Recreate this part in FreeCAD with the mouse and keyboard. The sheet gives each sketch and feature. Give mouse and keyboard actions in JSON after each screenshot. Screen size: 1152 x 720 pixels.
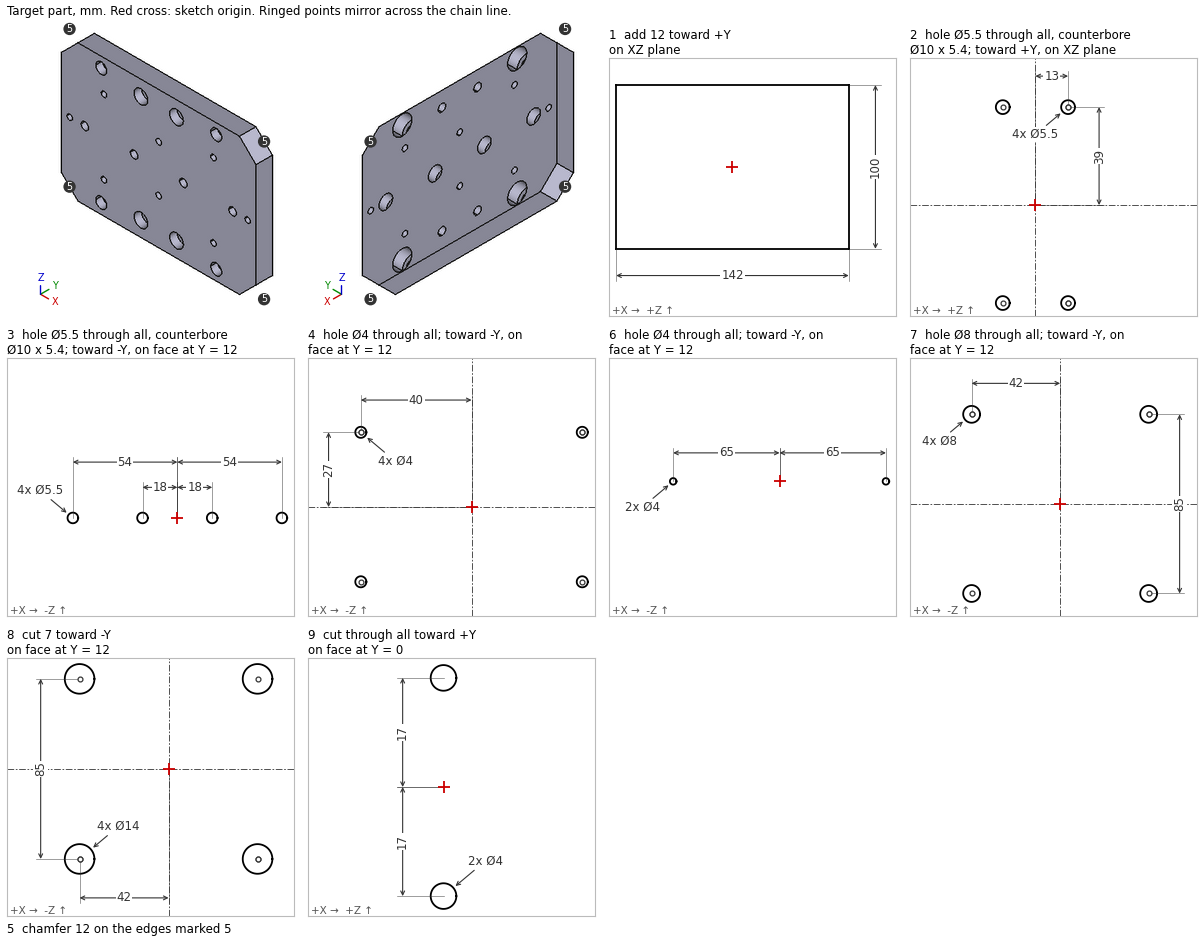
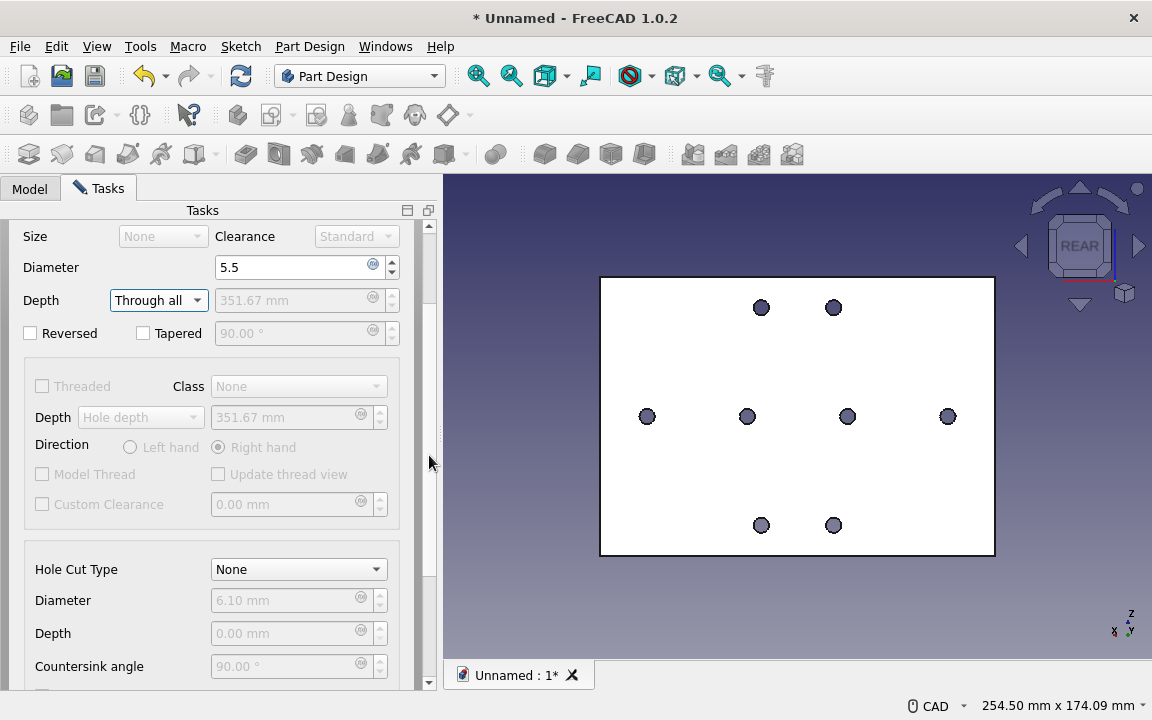
{"action": "left_click", "coordinate": [300, 570]}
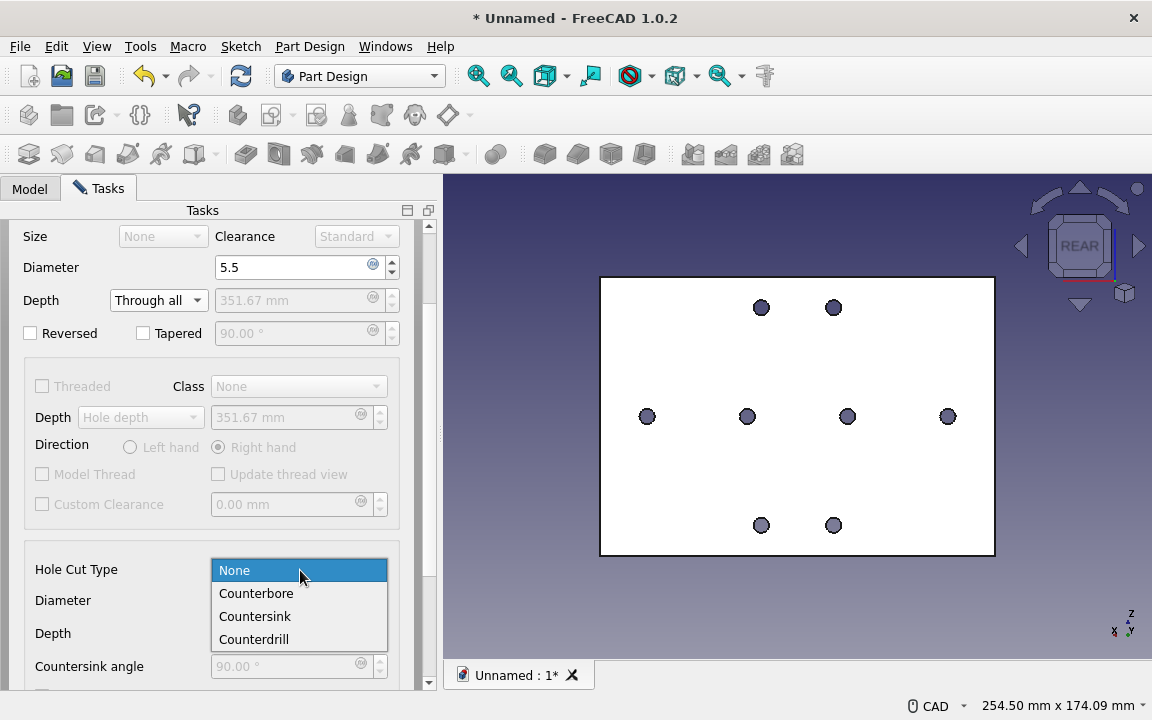
{"action": "left_click", "coordinate": [298, 594]}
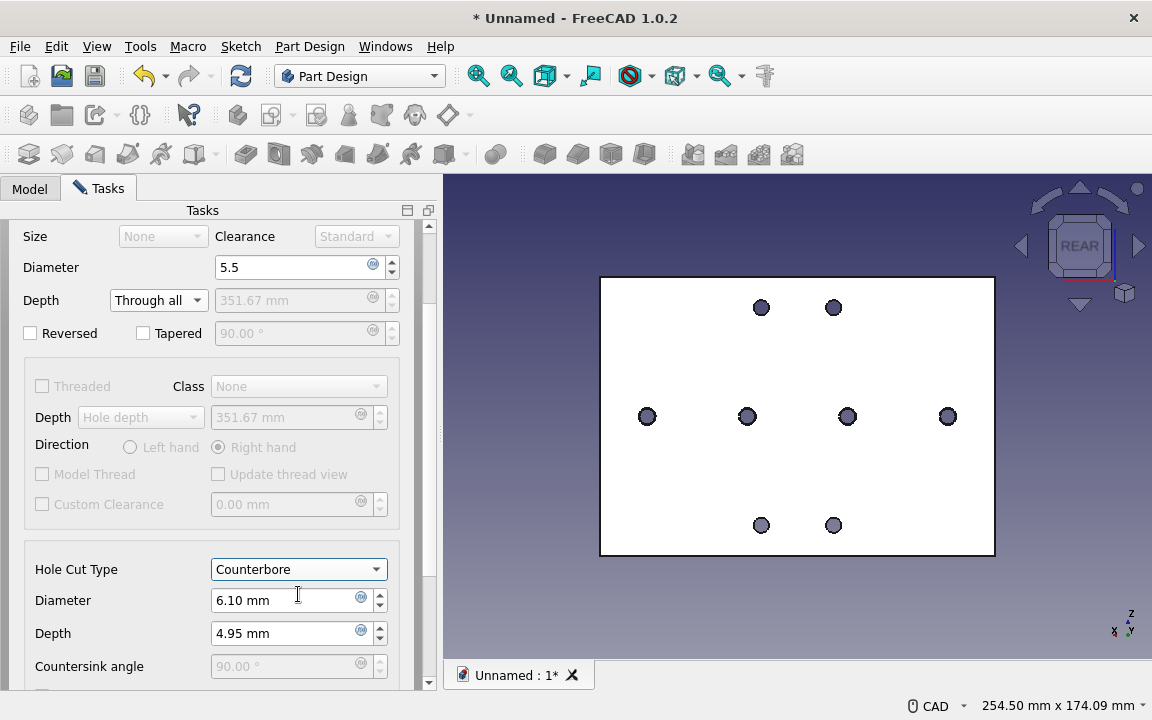
{"action": "triple_click", "coordinate": [292, 600]}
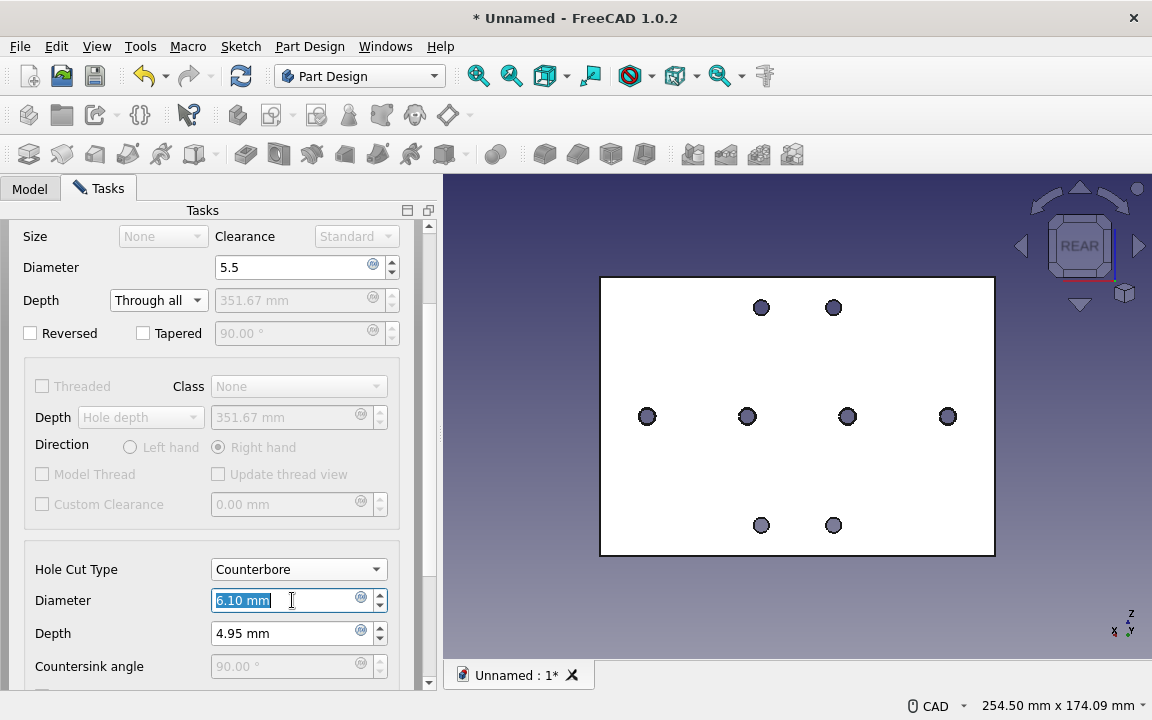
{"action": "type", "text": "10"}
{"action": "key", "text": "Tab"}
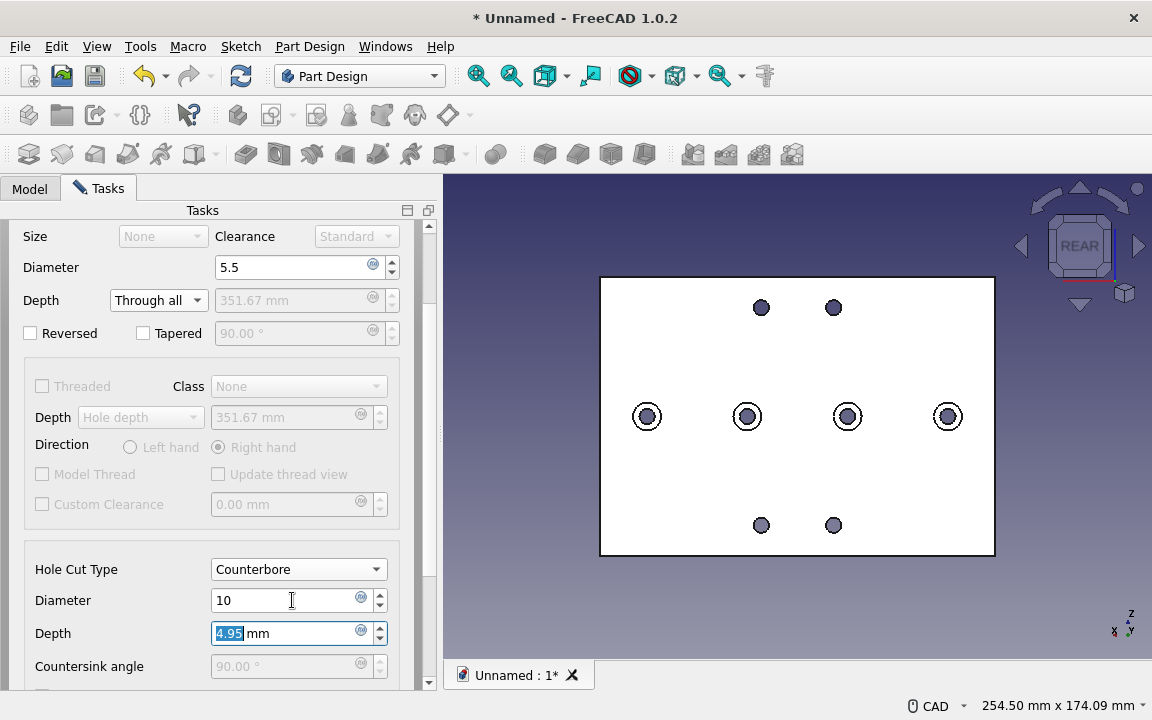
{"action": "type", "text": "5.4"}
{"action": "key", "text": "Tab"}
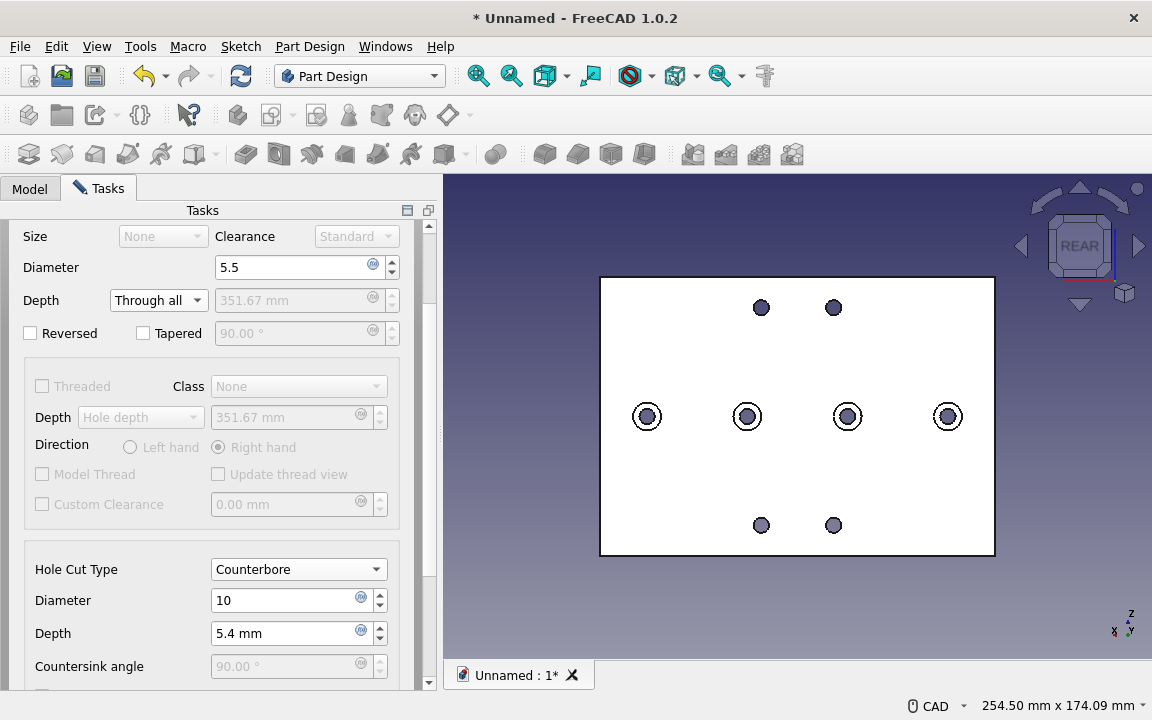
{"action": "scroll", "coordinate": [429, 455], "scroll_direction": "up", "scroll_amount": 3}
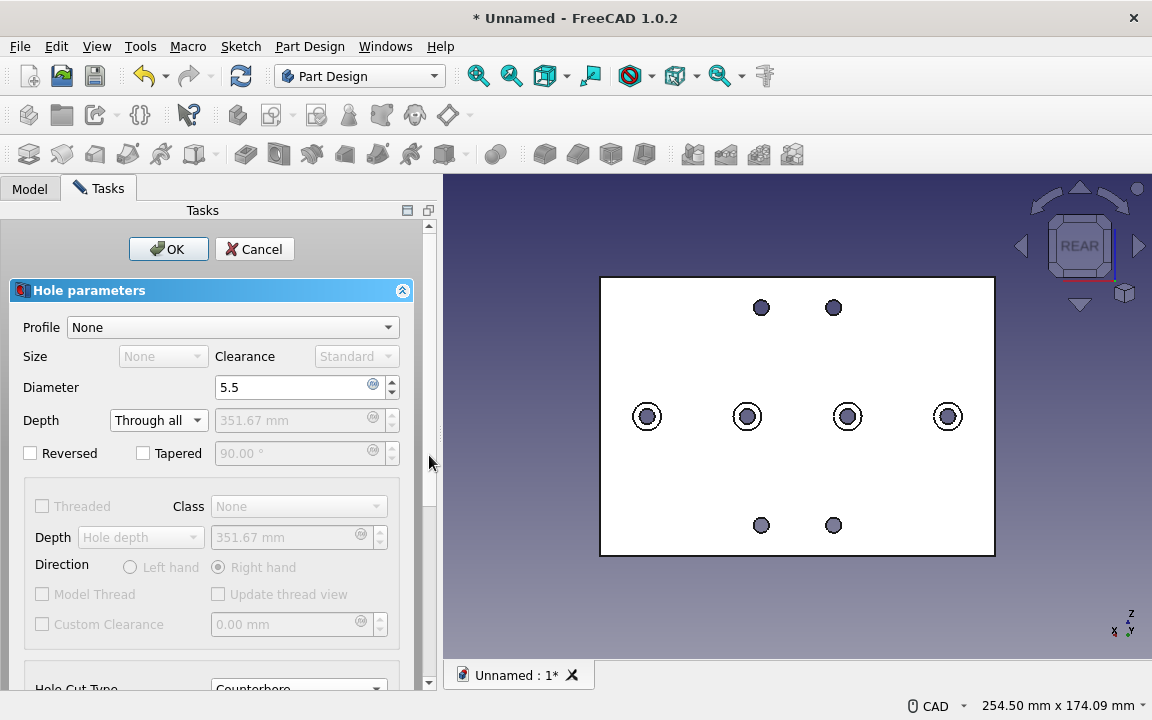
{"action": "left_click", "coordinate": [169, 249]}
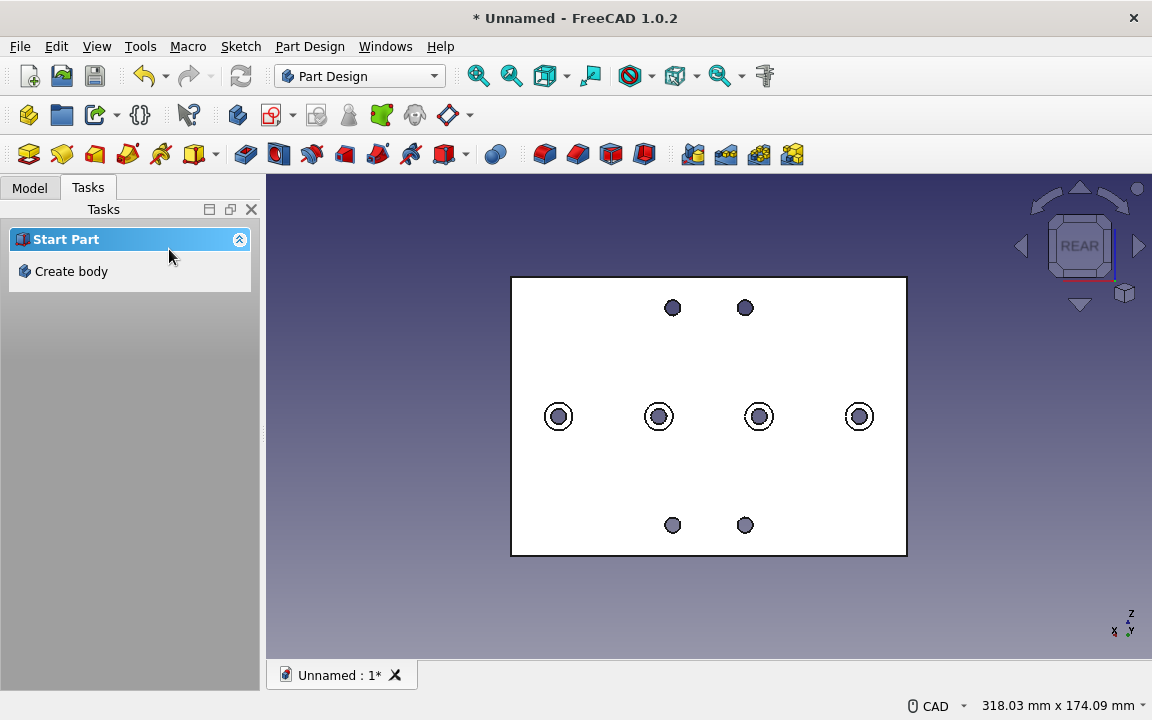
{"action": "left_click", "coordinate": [596, 336]}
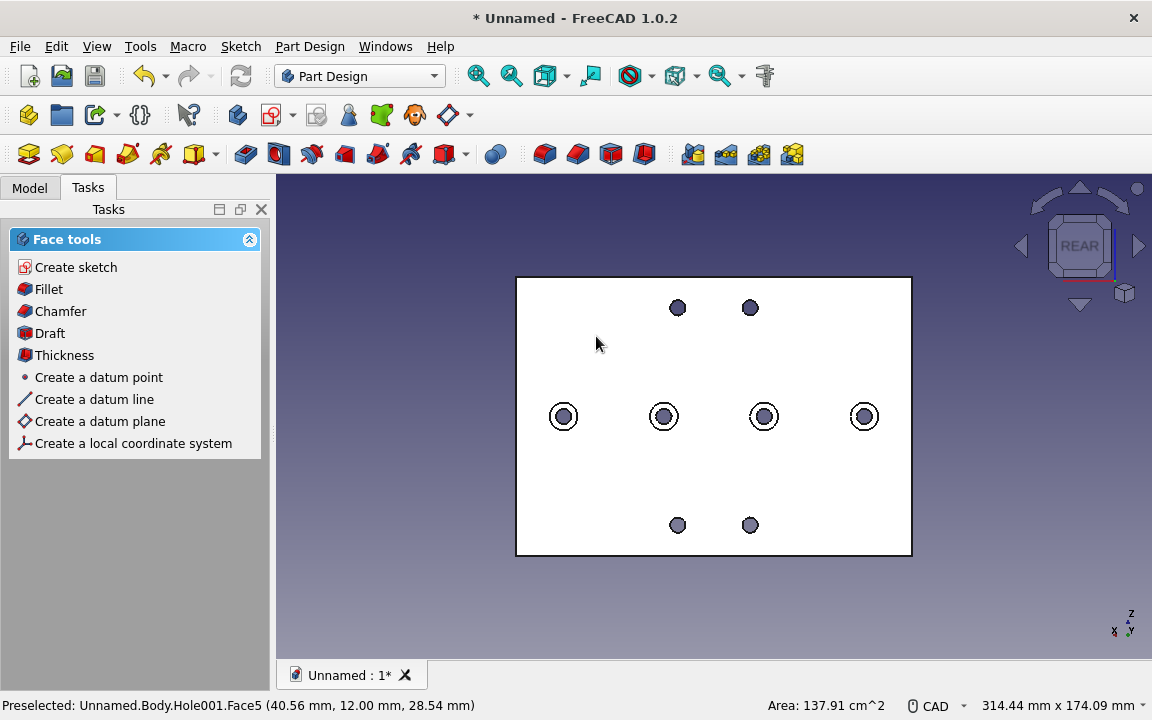
{"action": "left_click", "coordinate": [270, 116]}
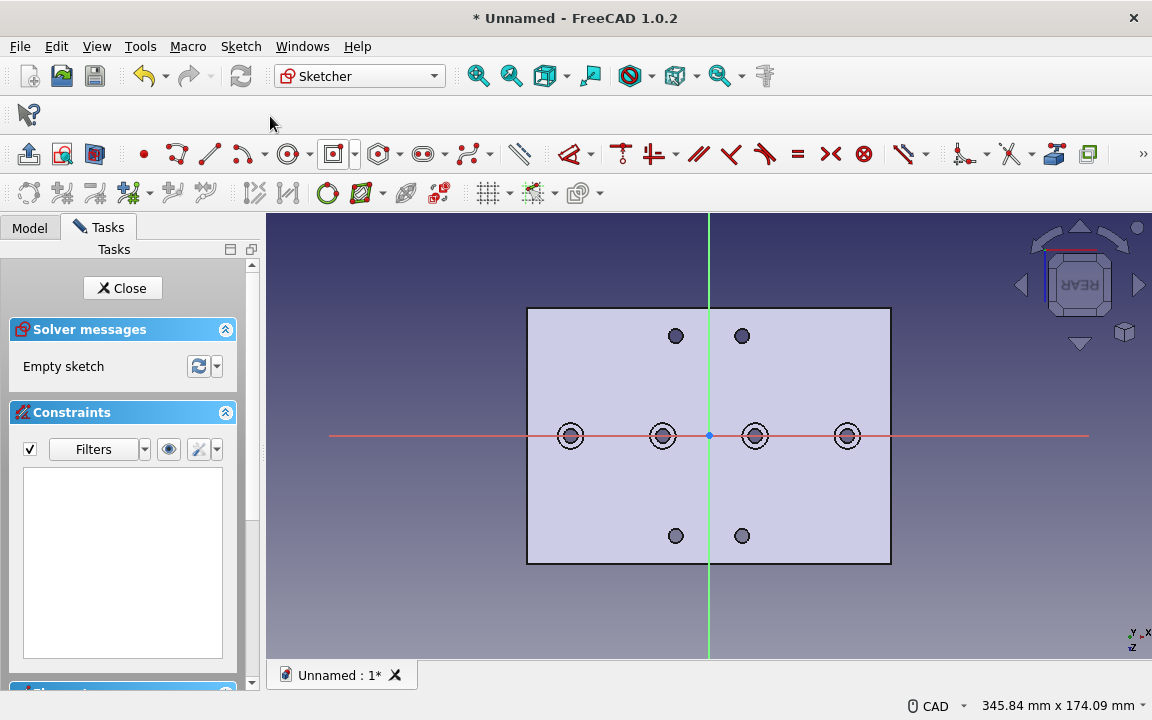
{"action": "scroll", "coordinate": [792, 436], "scroll_direction": "up", "scroll_amount": 3}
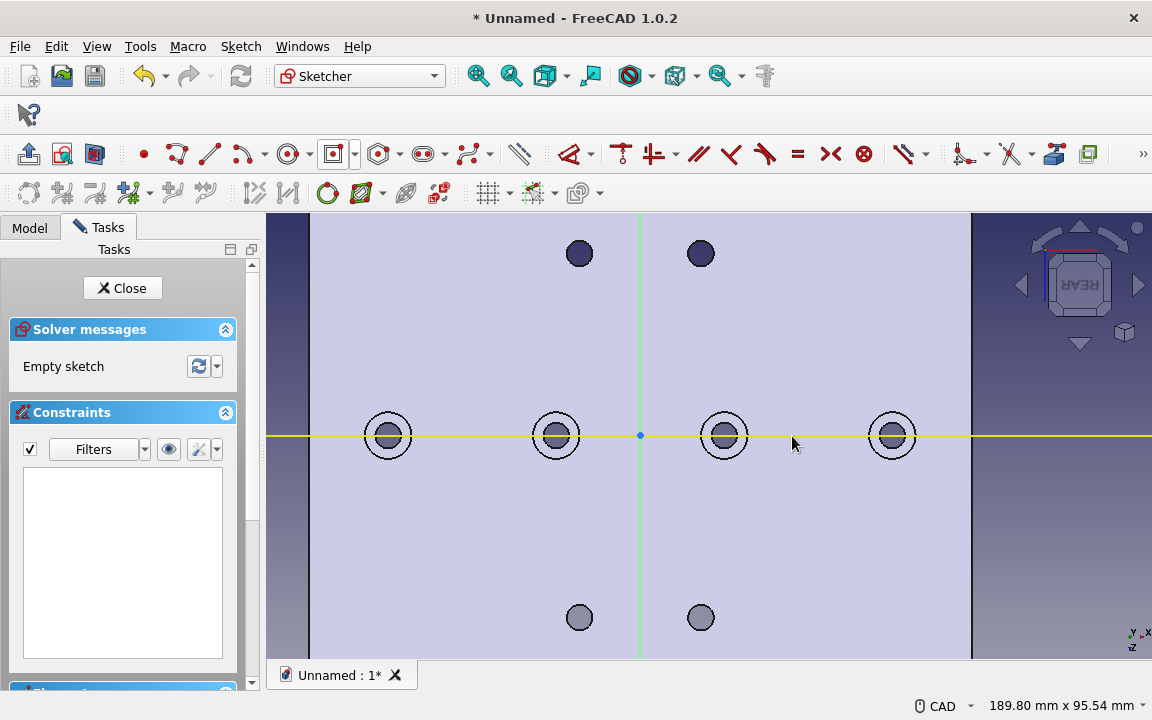
{"action": "left_click", "coordinate": [288, 154]}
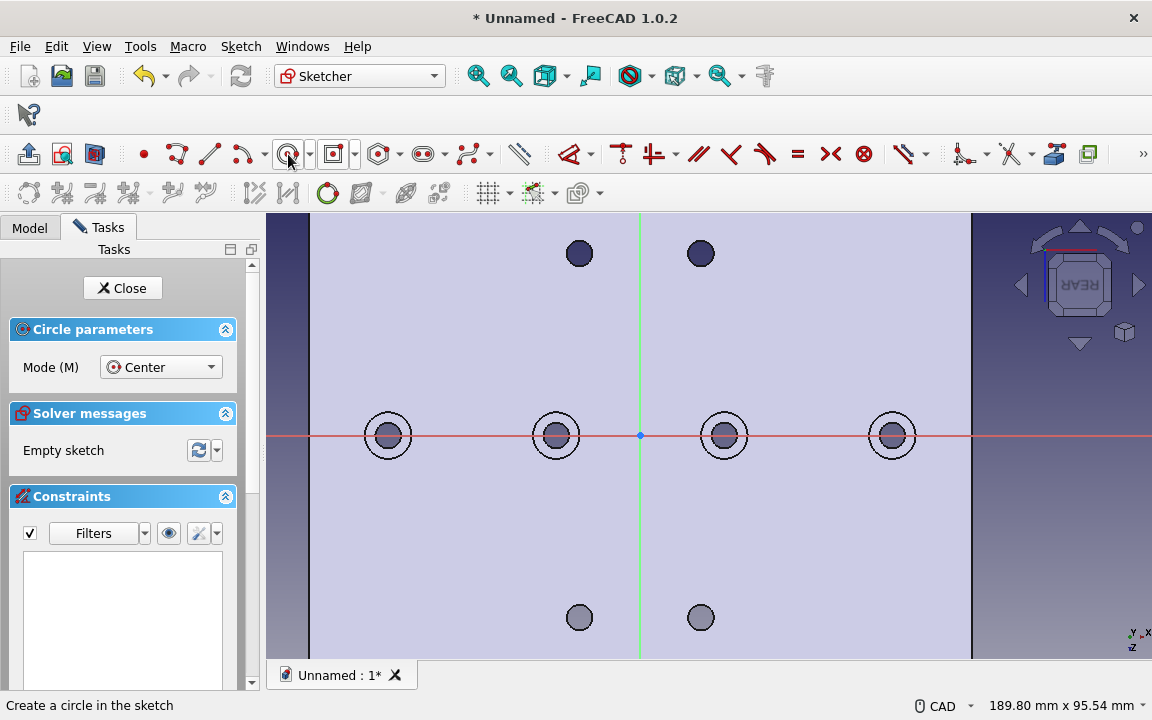
{"action": "scroll", "coordinate": [454, 310], "scroll_direction": "up", "scroll_amount": 5}